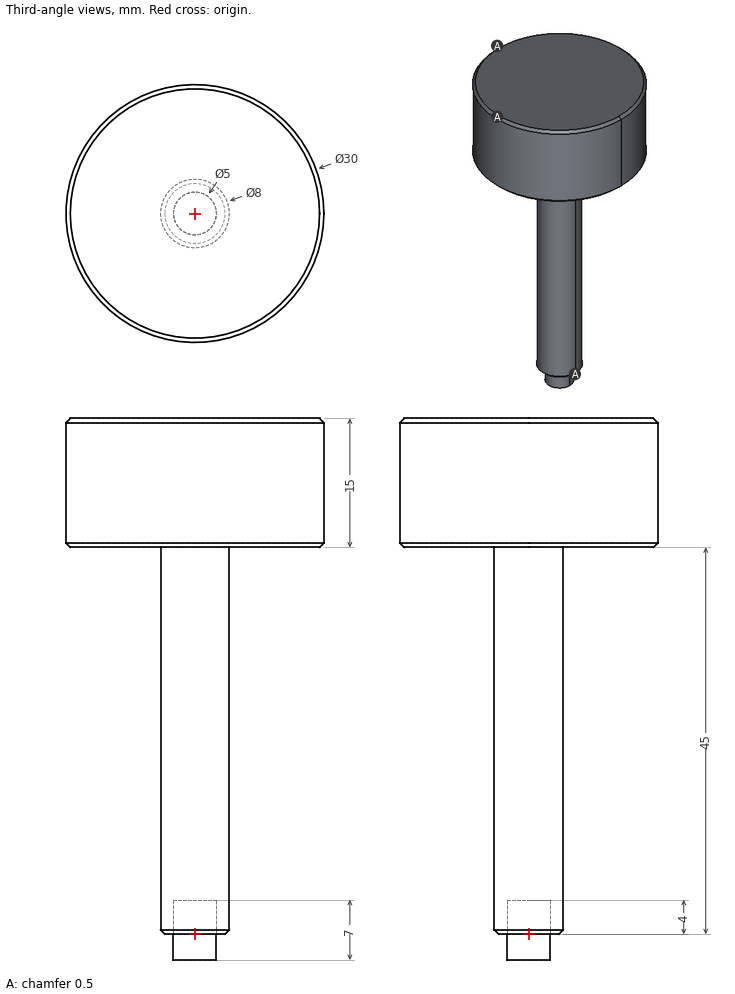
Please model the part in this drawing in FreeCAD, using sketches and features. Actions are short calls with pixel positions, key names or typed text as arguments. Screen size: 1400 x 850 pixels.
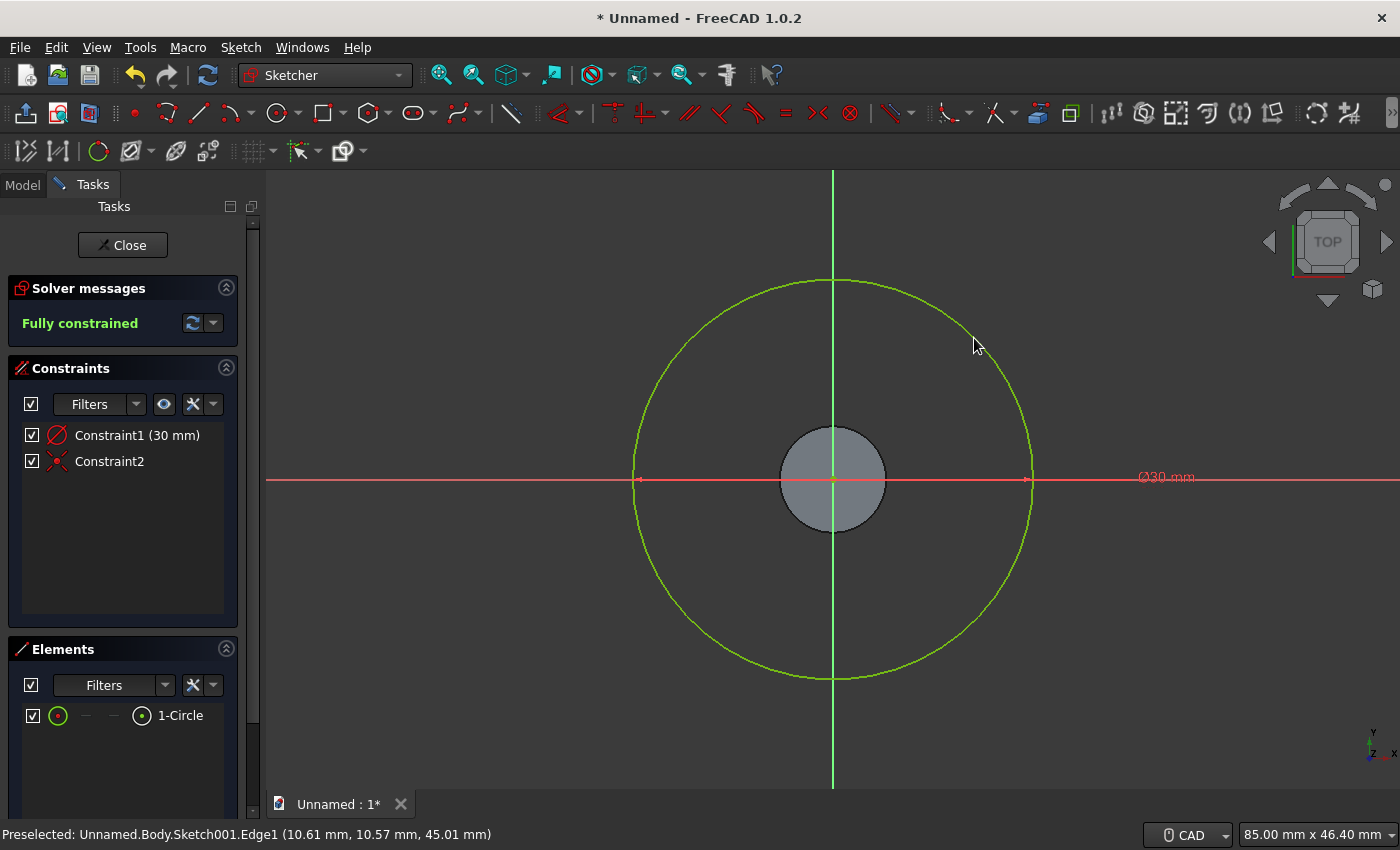
click(123, 245)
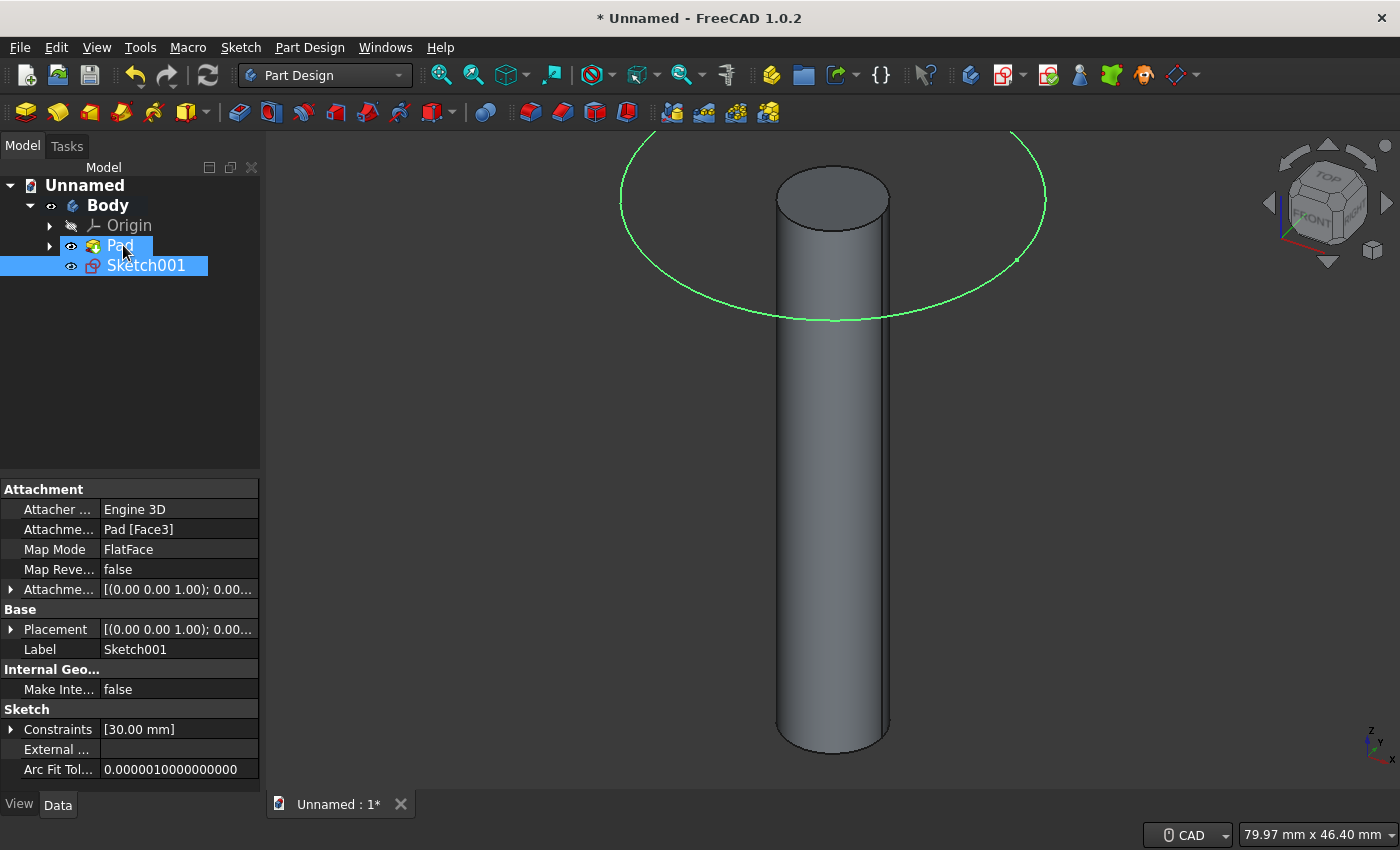
click(26, 112)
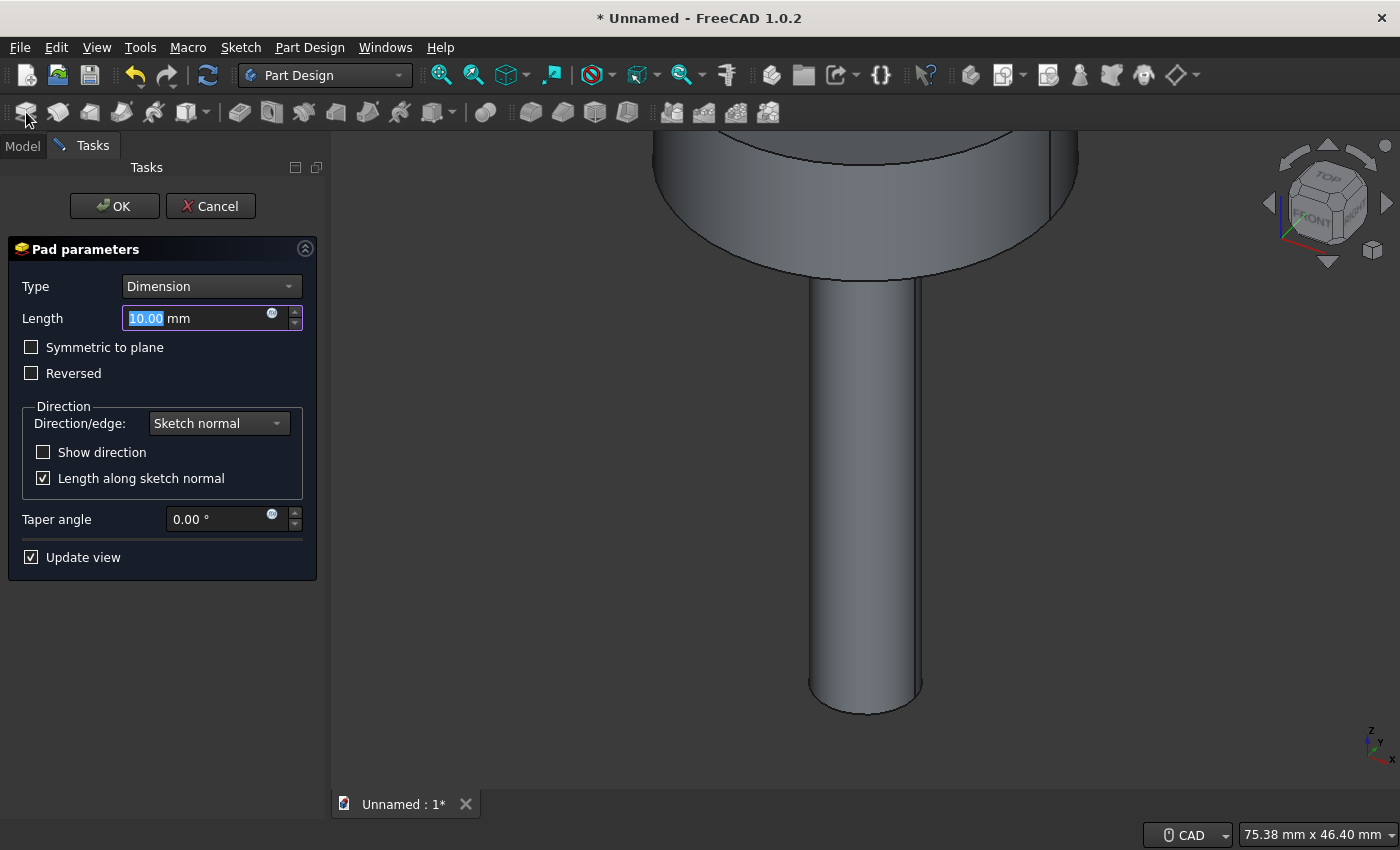
text(15)
key(Tab)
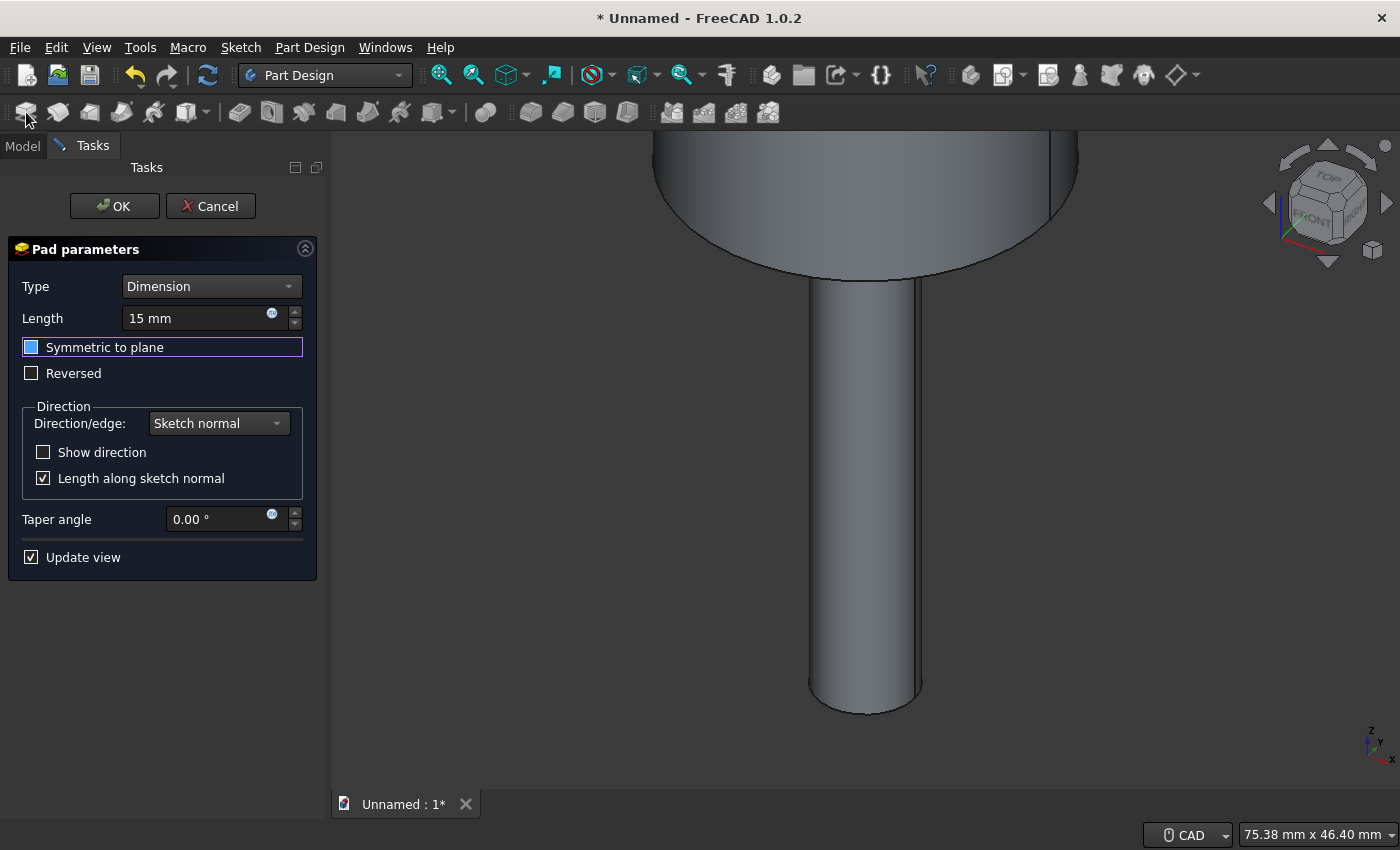
click(115, 206)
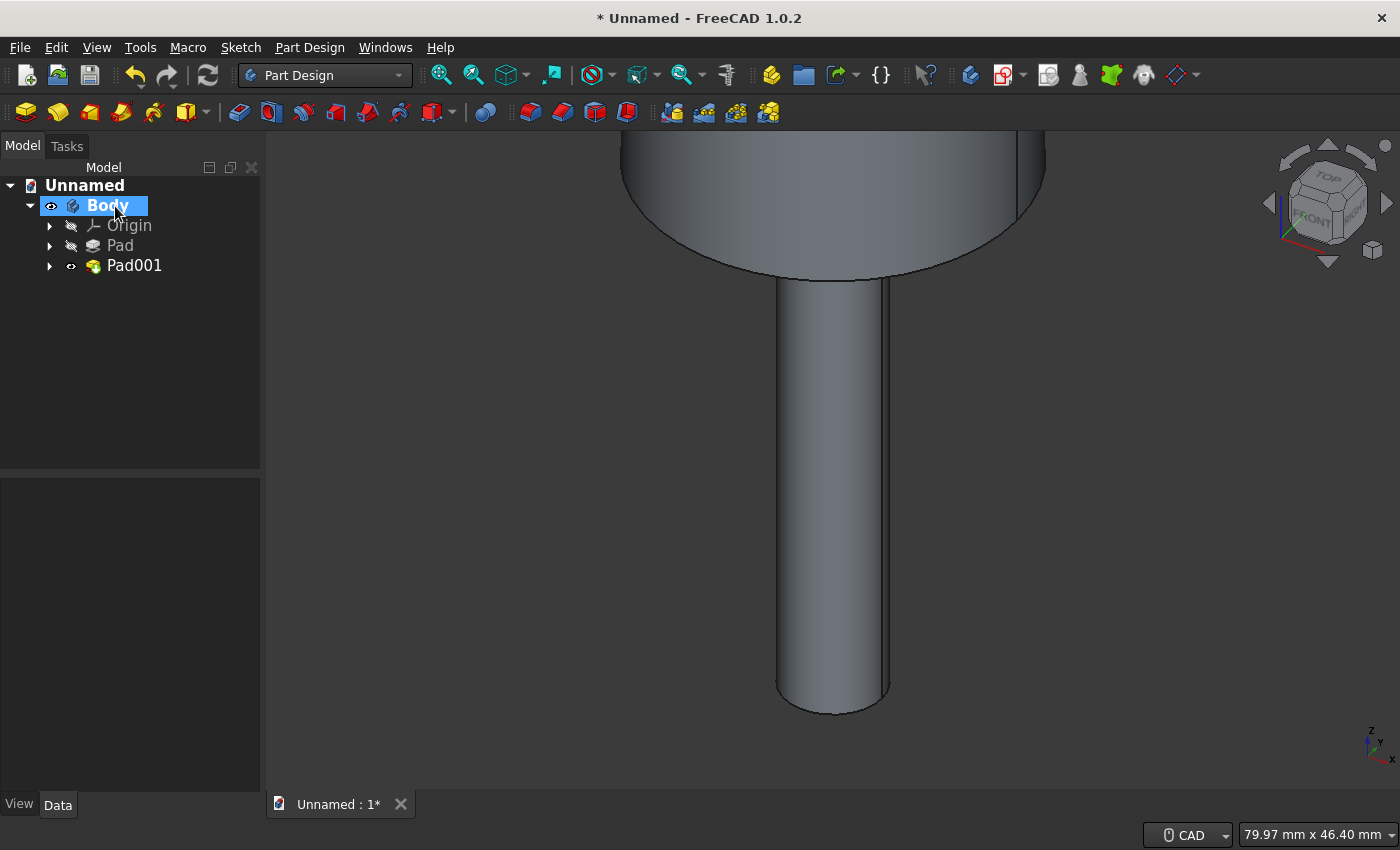
click(442, 76)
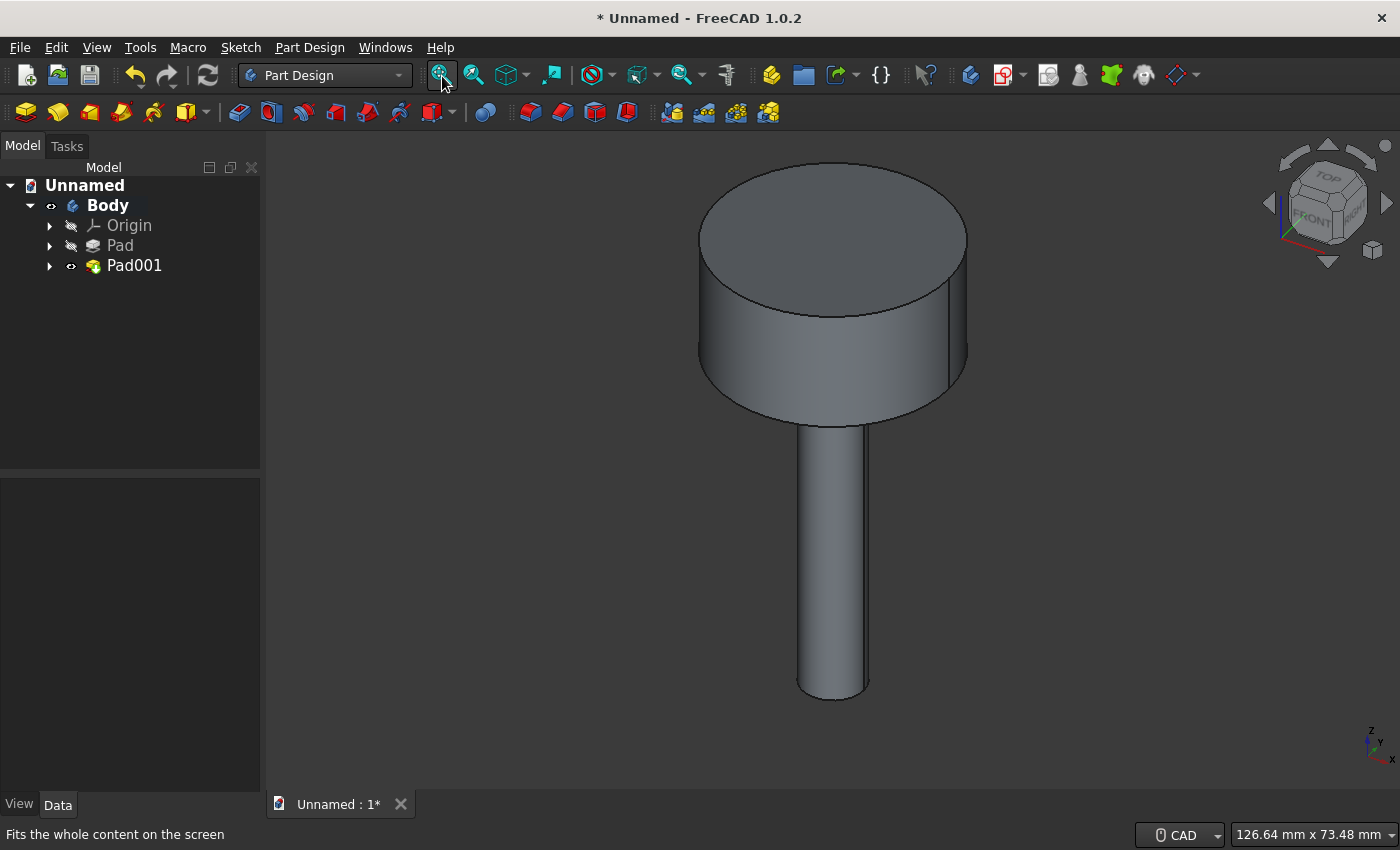
click(1004, 76)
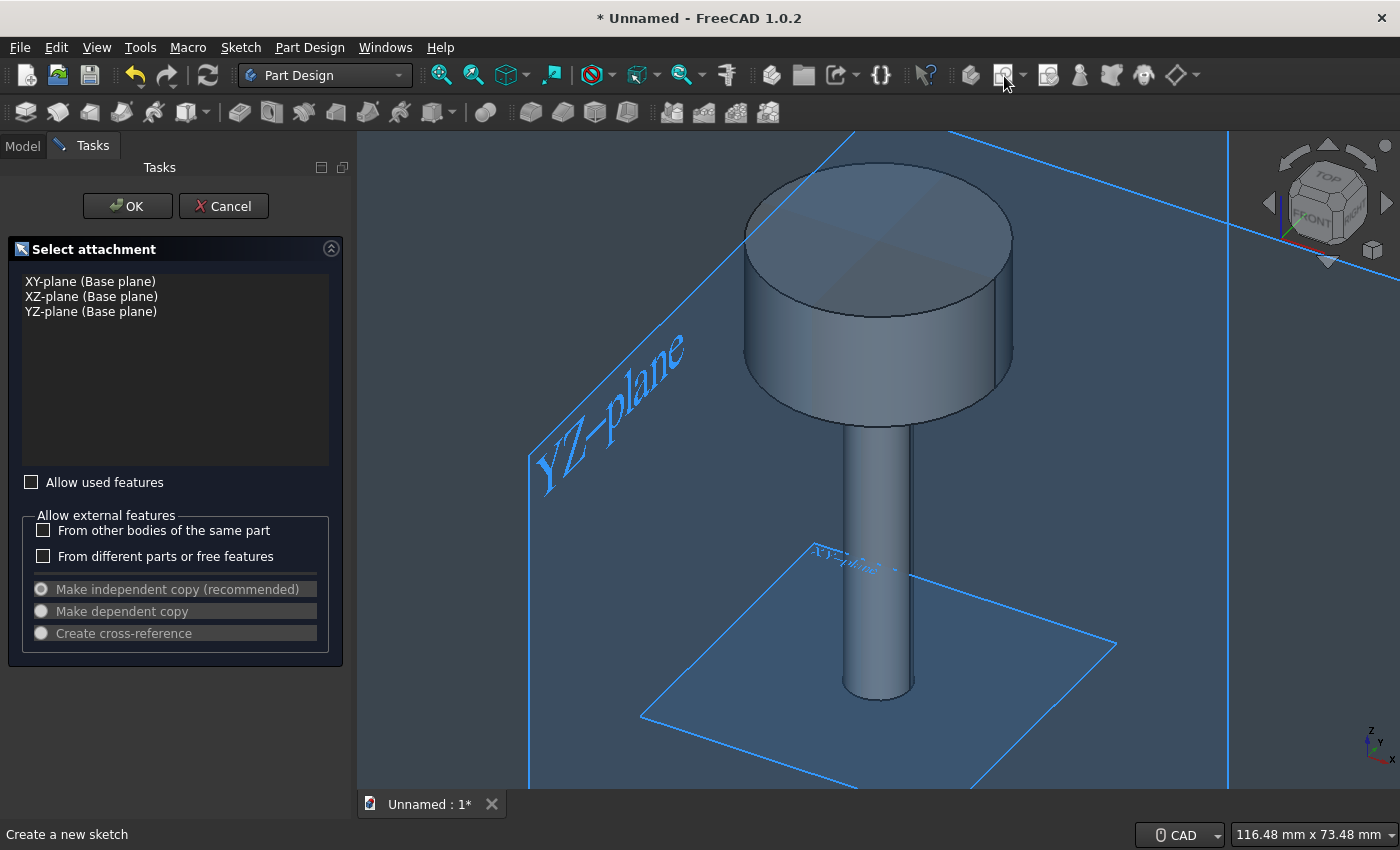
click(82, 282)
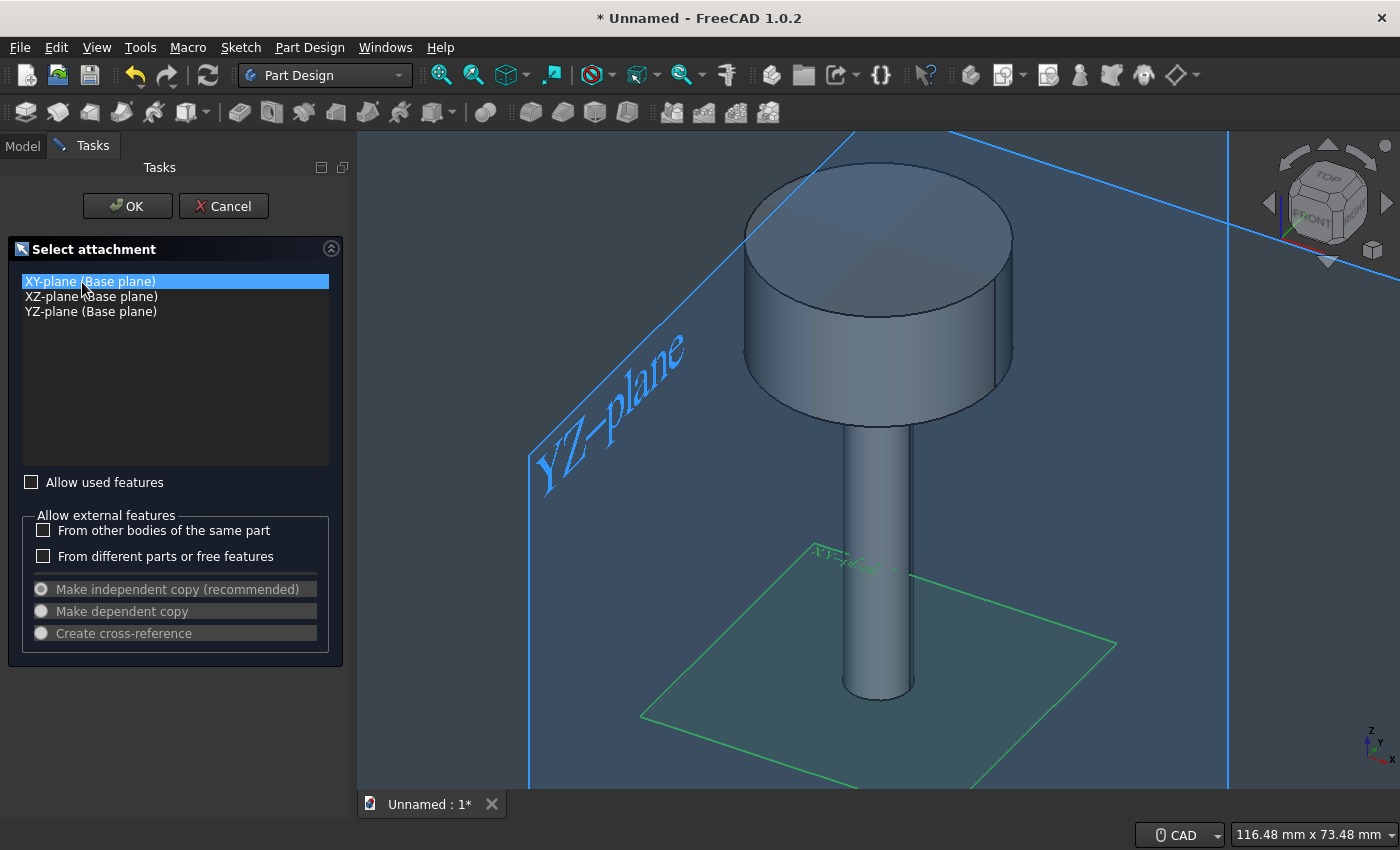
click(128, 206)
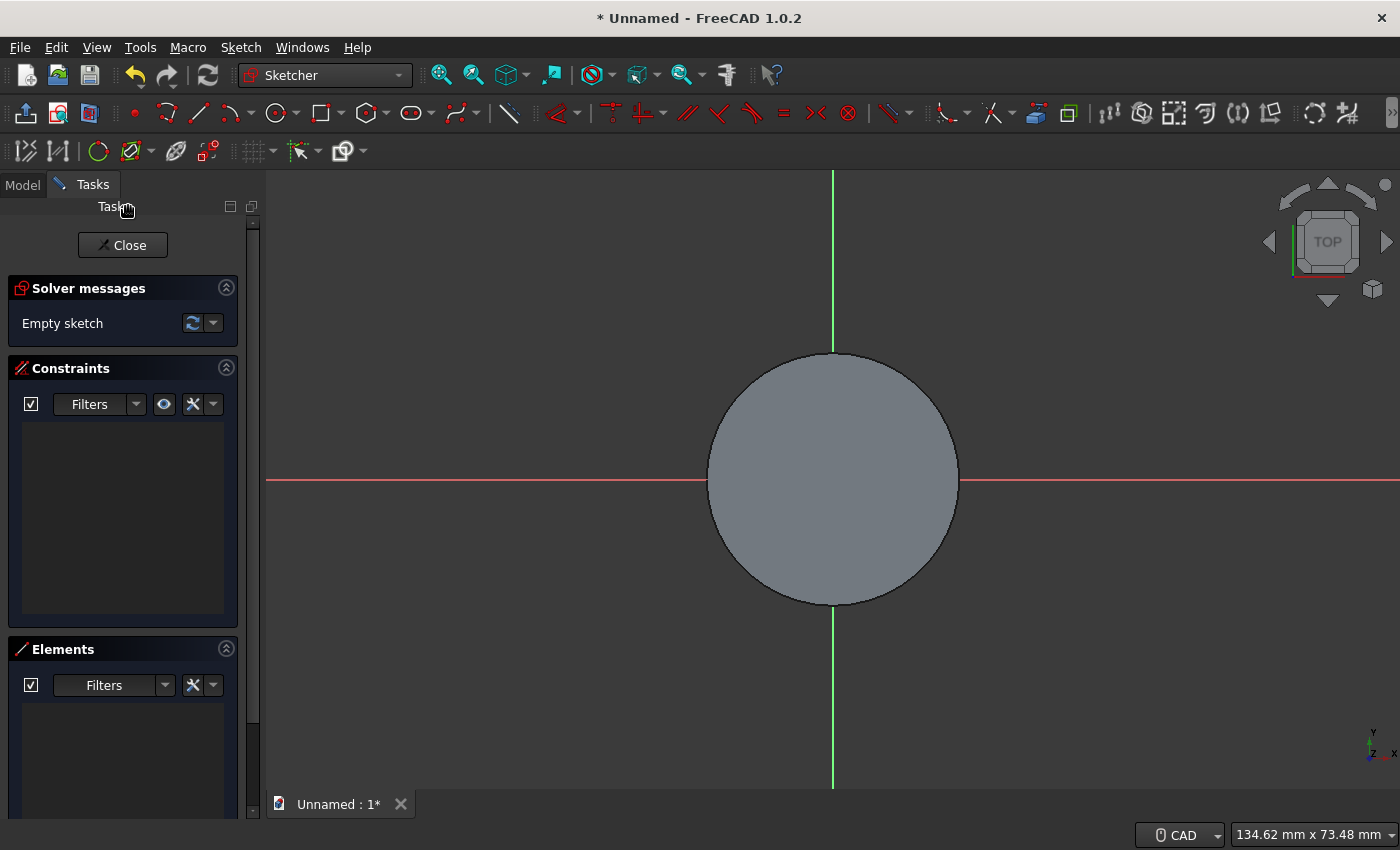
click(90, 114)